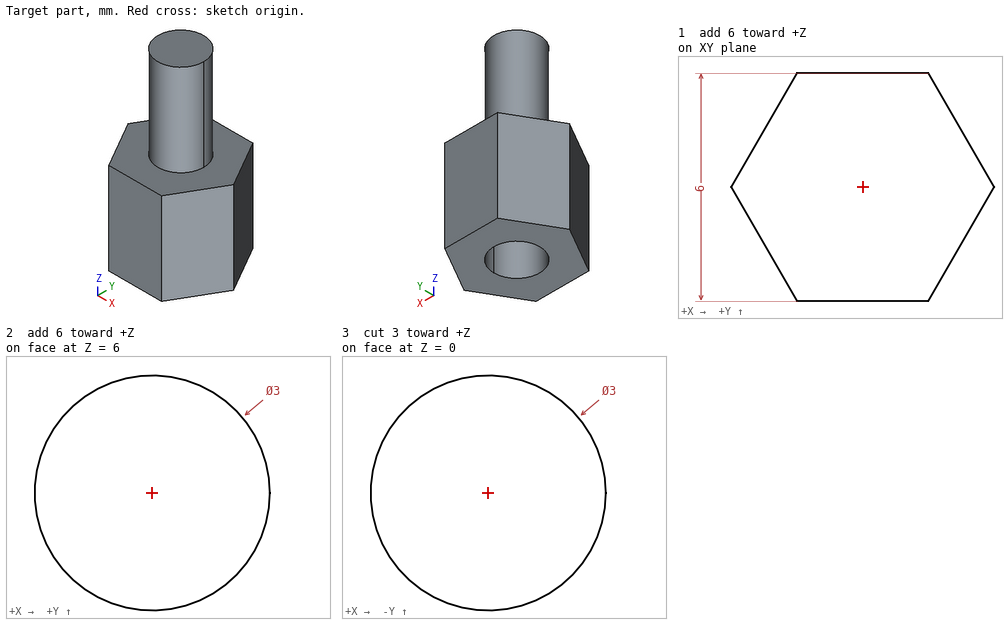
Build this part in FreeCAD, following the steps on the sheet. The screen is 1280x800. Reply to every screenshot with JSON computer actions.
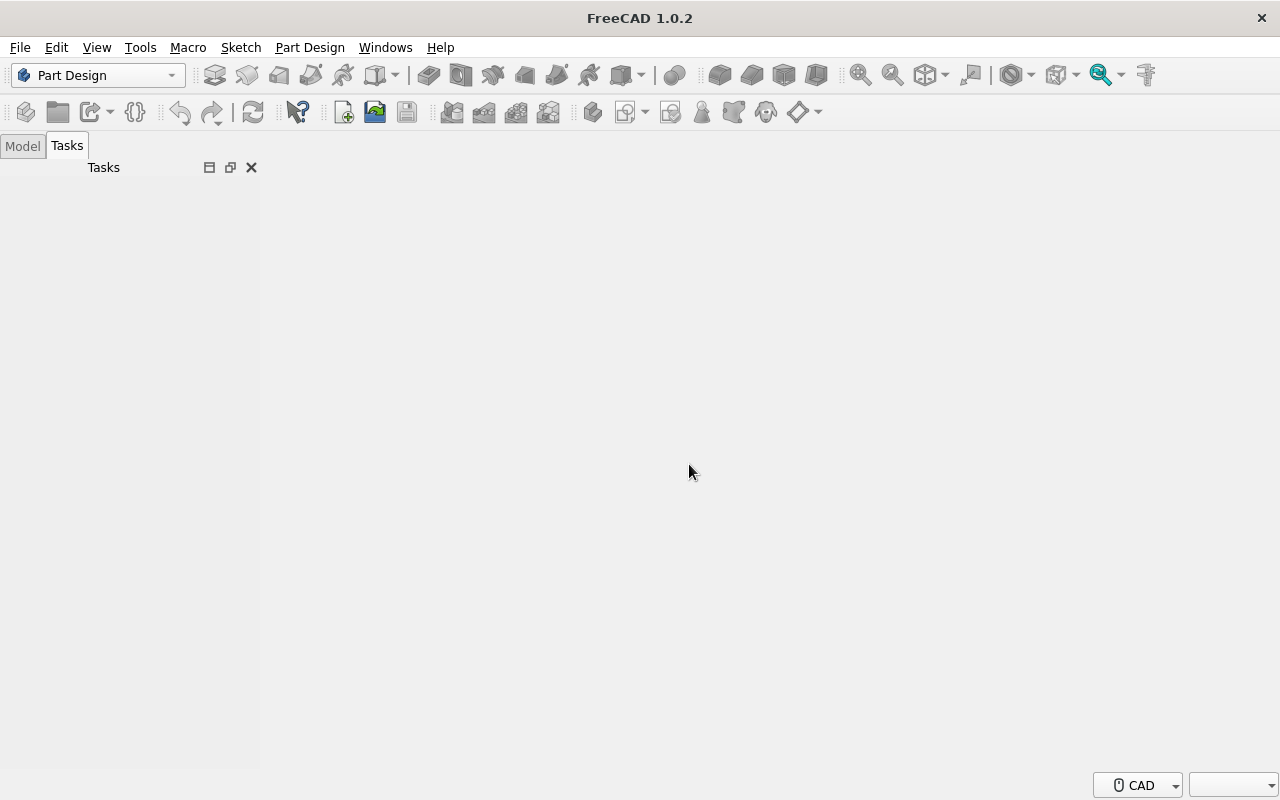
{"action": "left_click", "coordinate": [344, 112]}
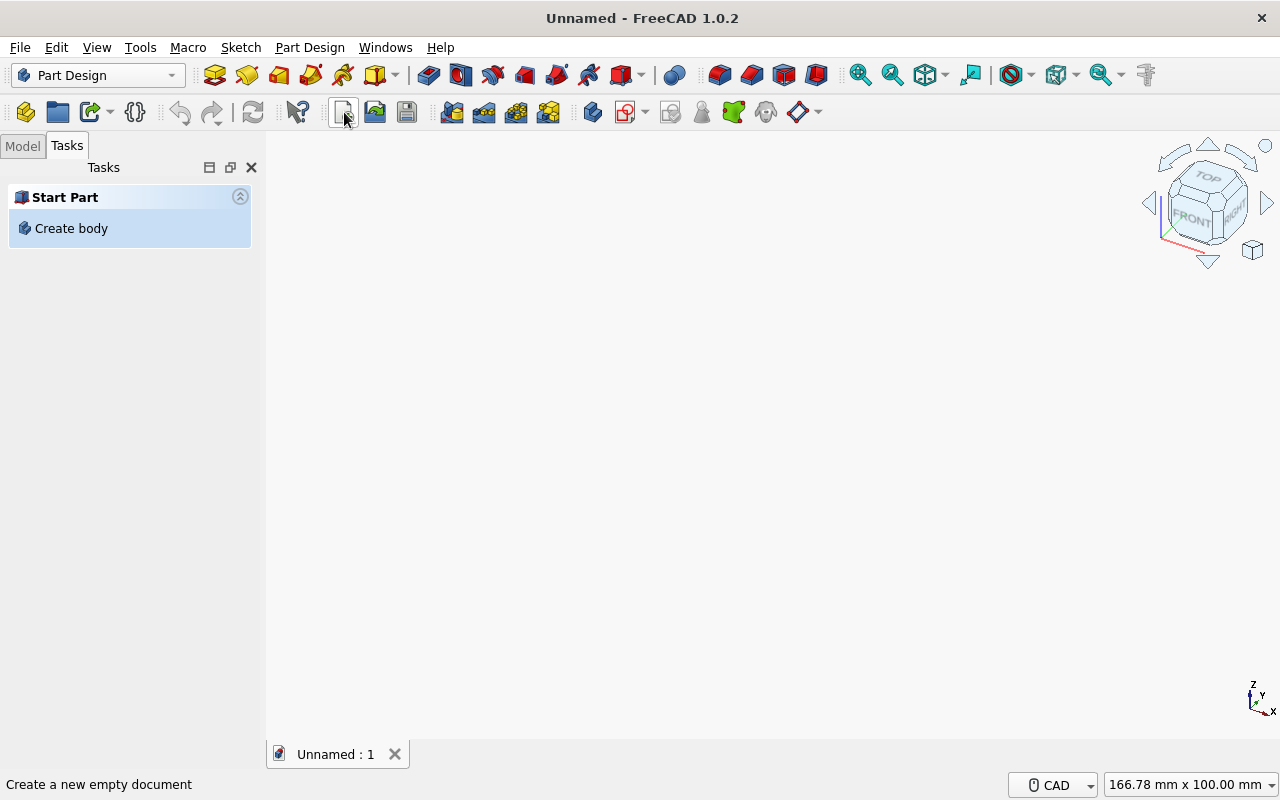
{"action": "left_click", "coordinate": [626, 112]}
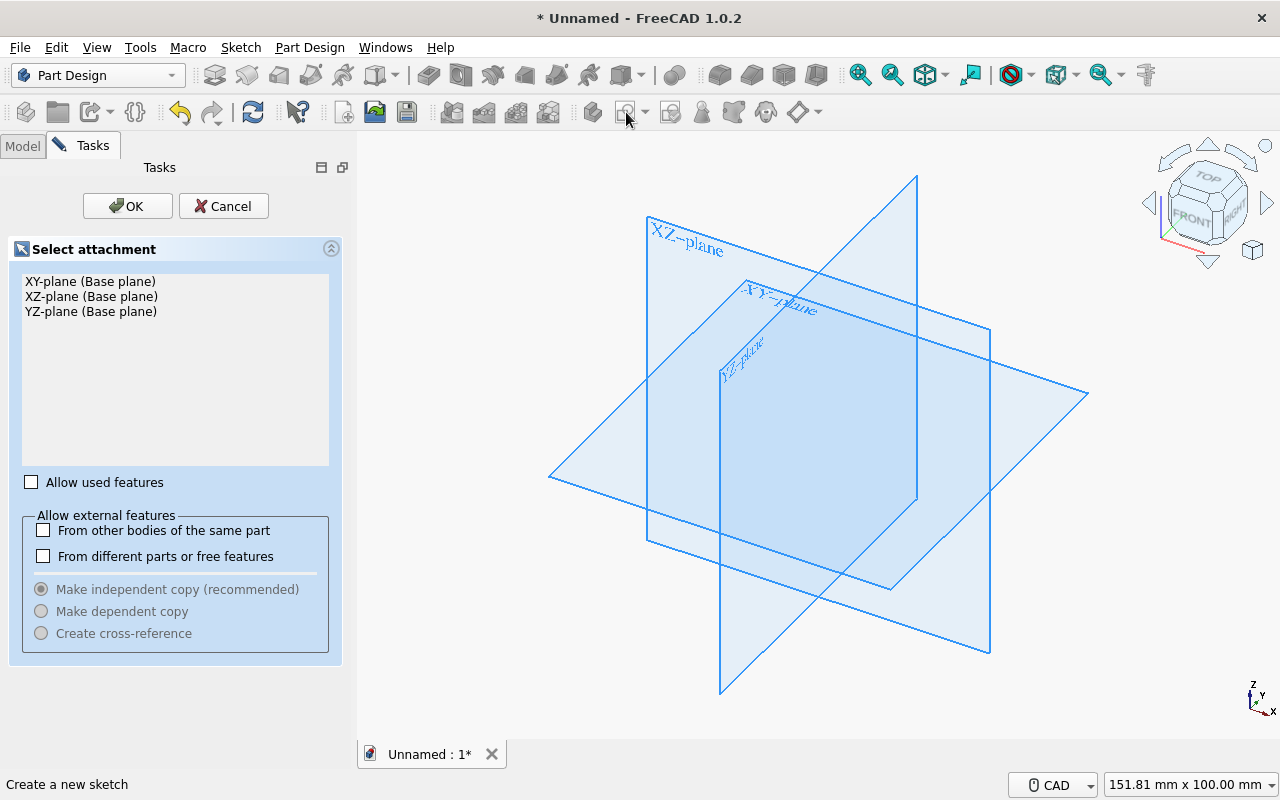
{"action": "left_click", "coordinate": [82, 282]}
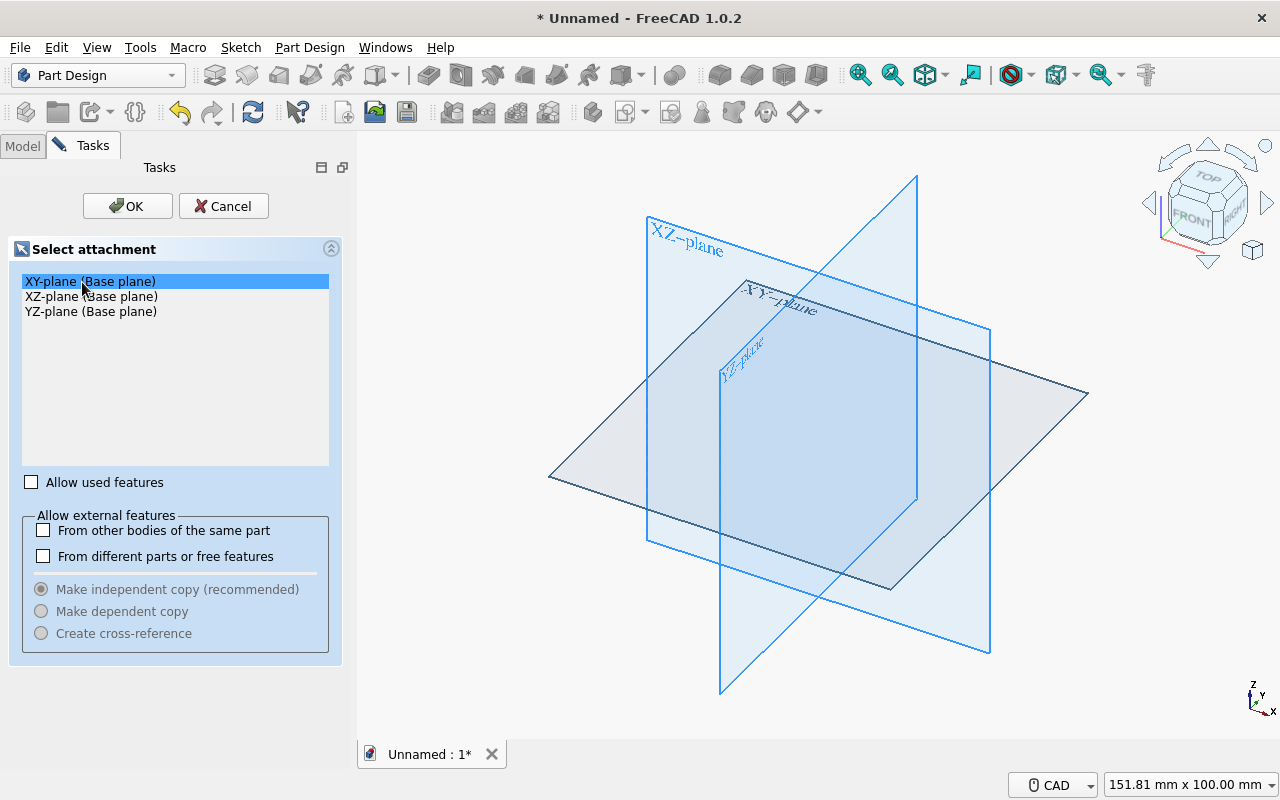
{"action": "left_click", "coordinate": [128, 206]}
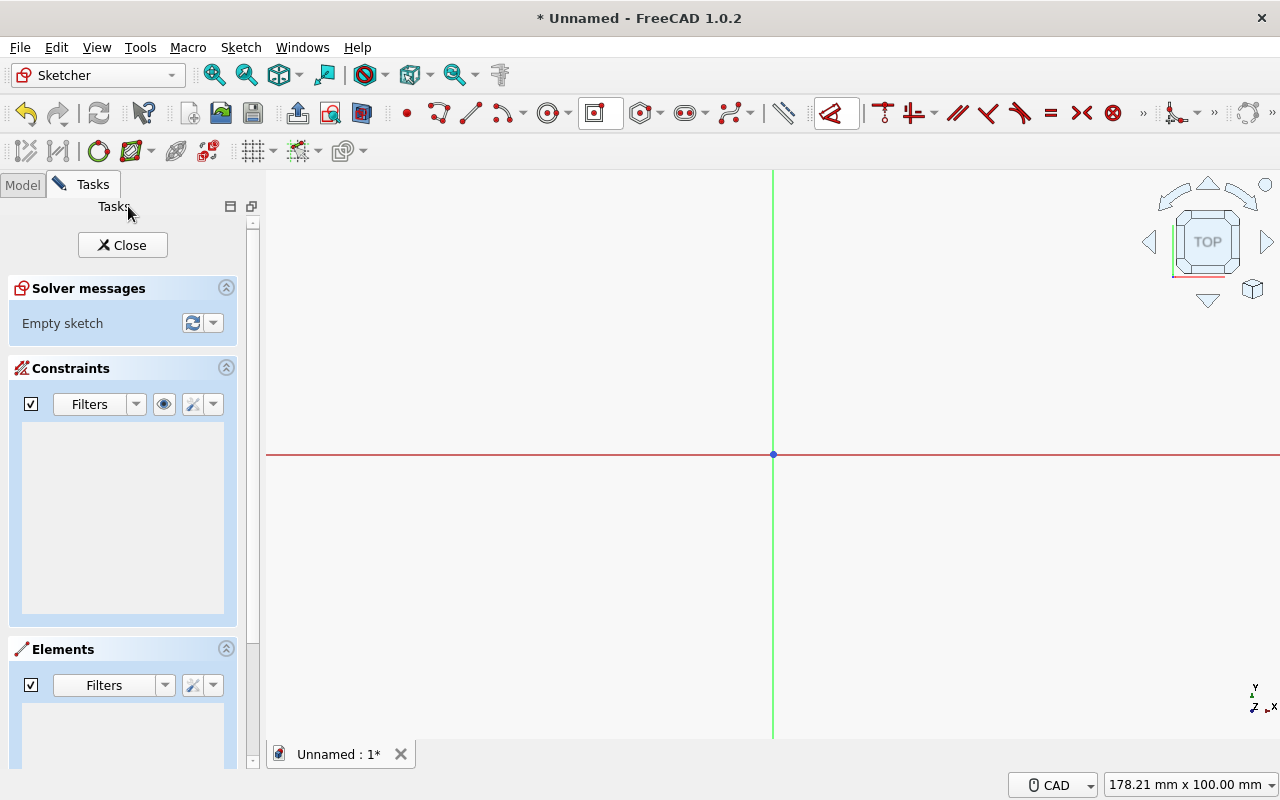
{"action": "scroll", "coordinate": [780, 455], "scroll_direction": "up", "scroll_amount": 12}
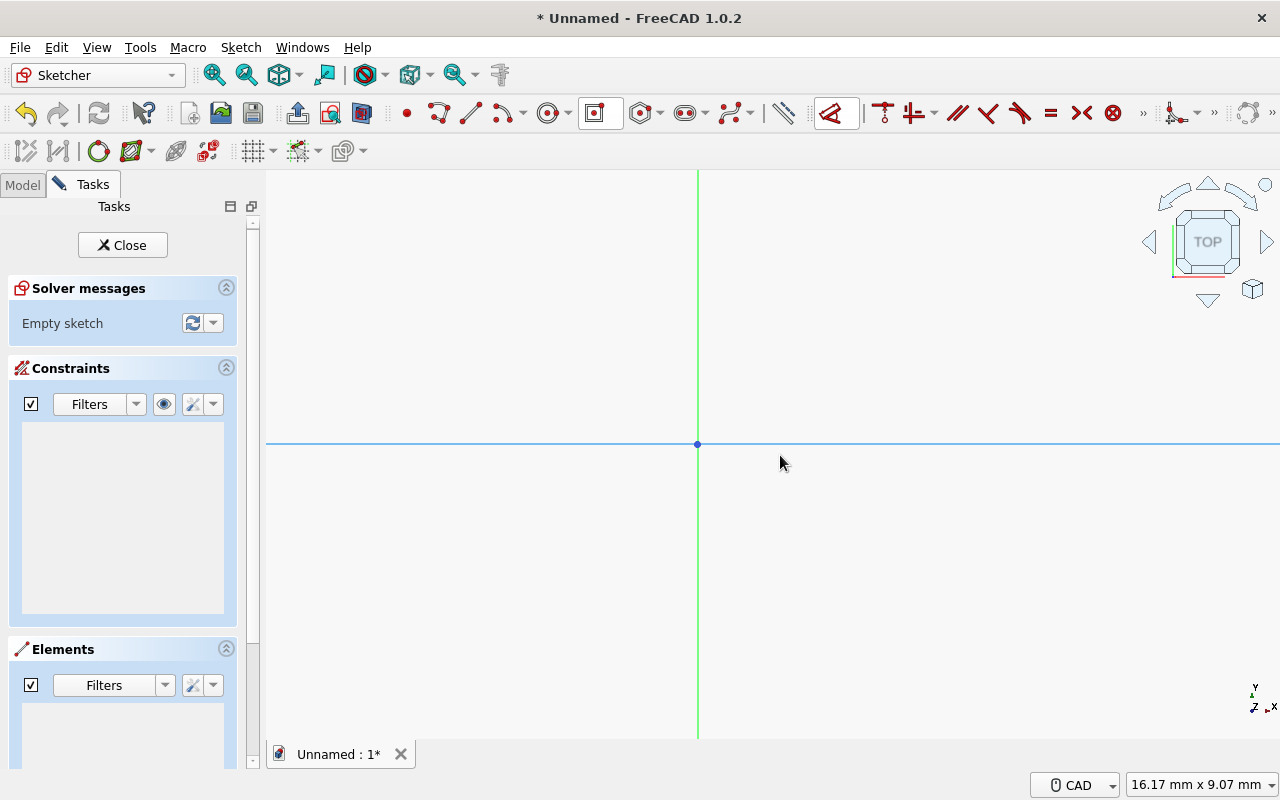
{"action": "key", "text": "g p 6"}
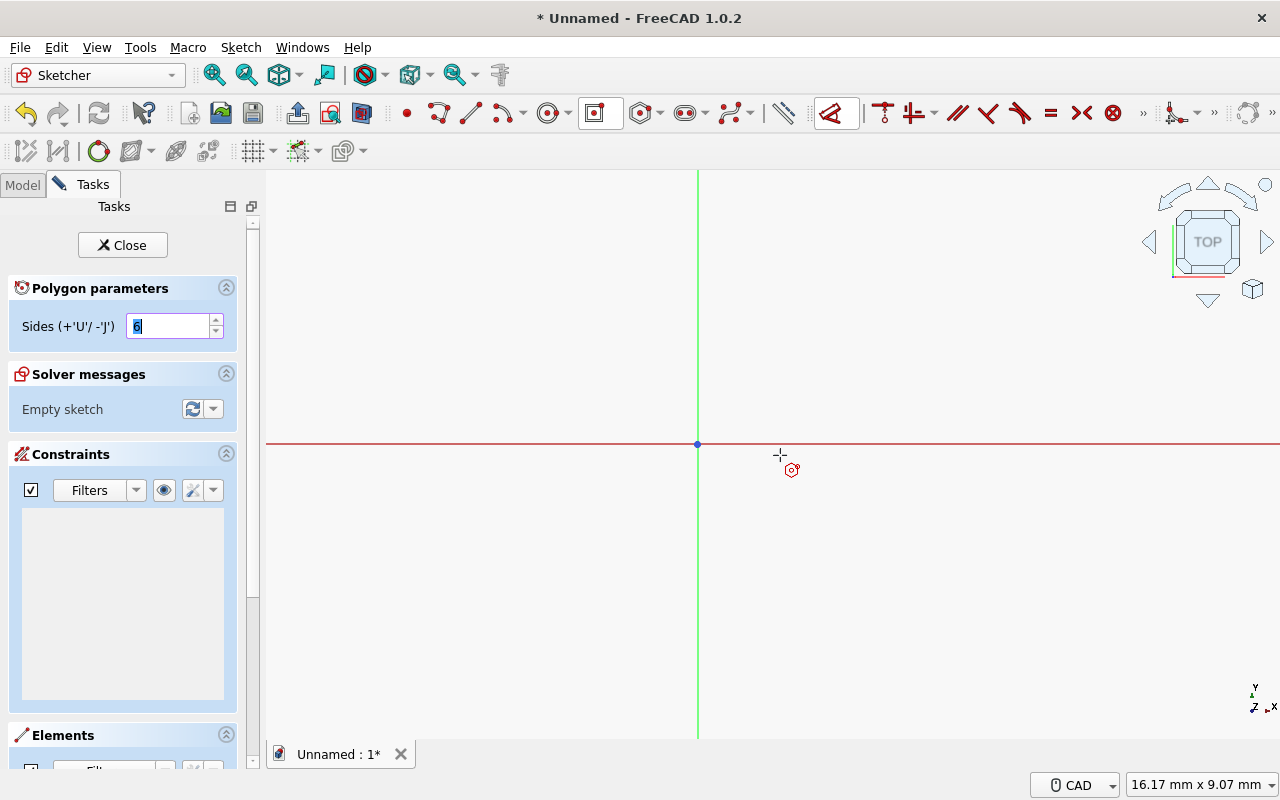
{"action": "left_click", "coordinate": [698, 444]}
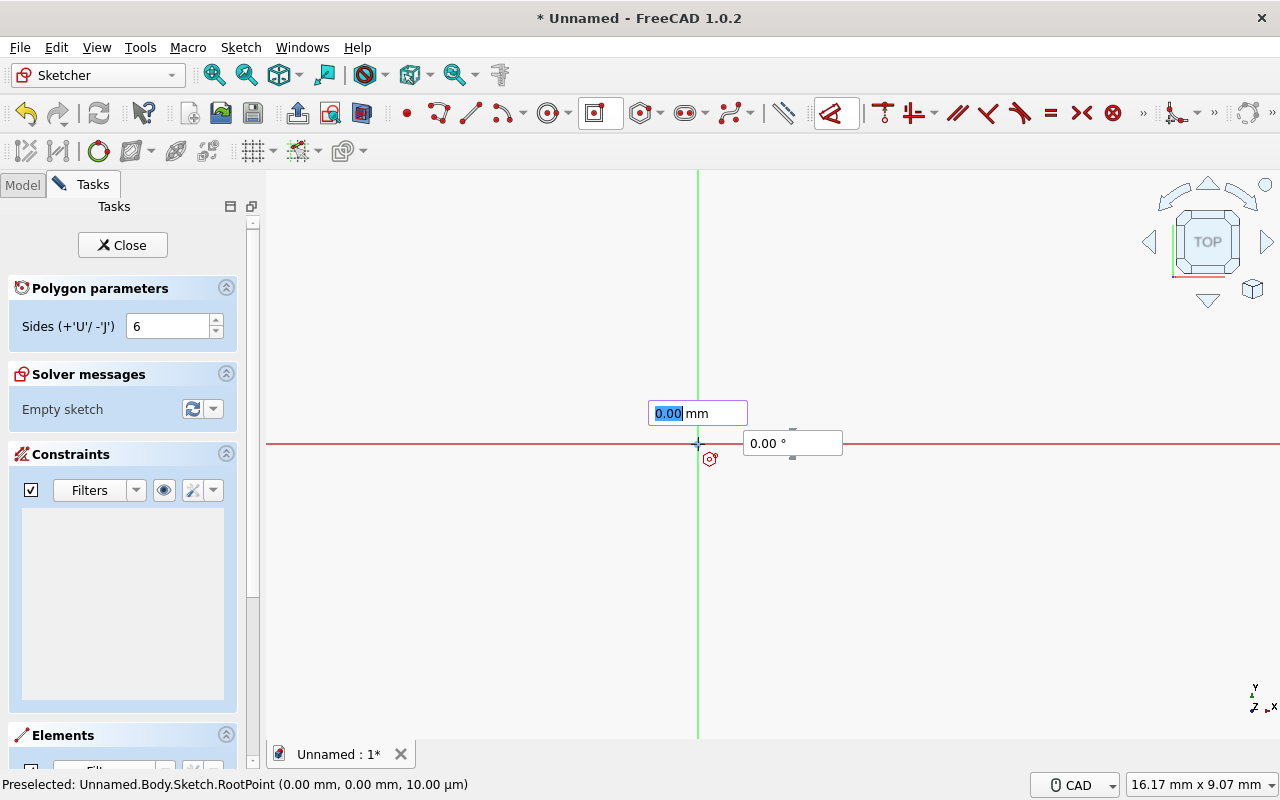
{"action": "left_click", "coordinate": [915, 444]}
{"action": "right_click", "coordinate": [915, 444]}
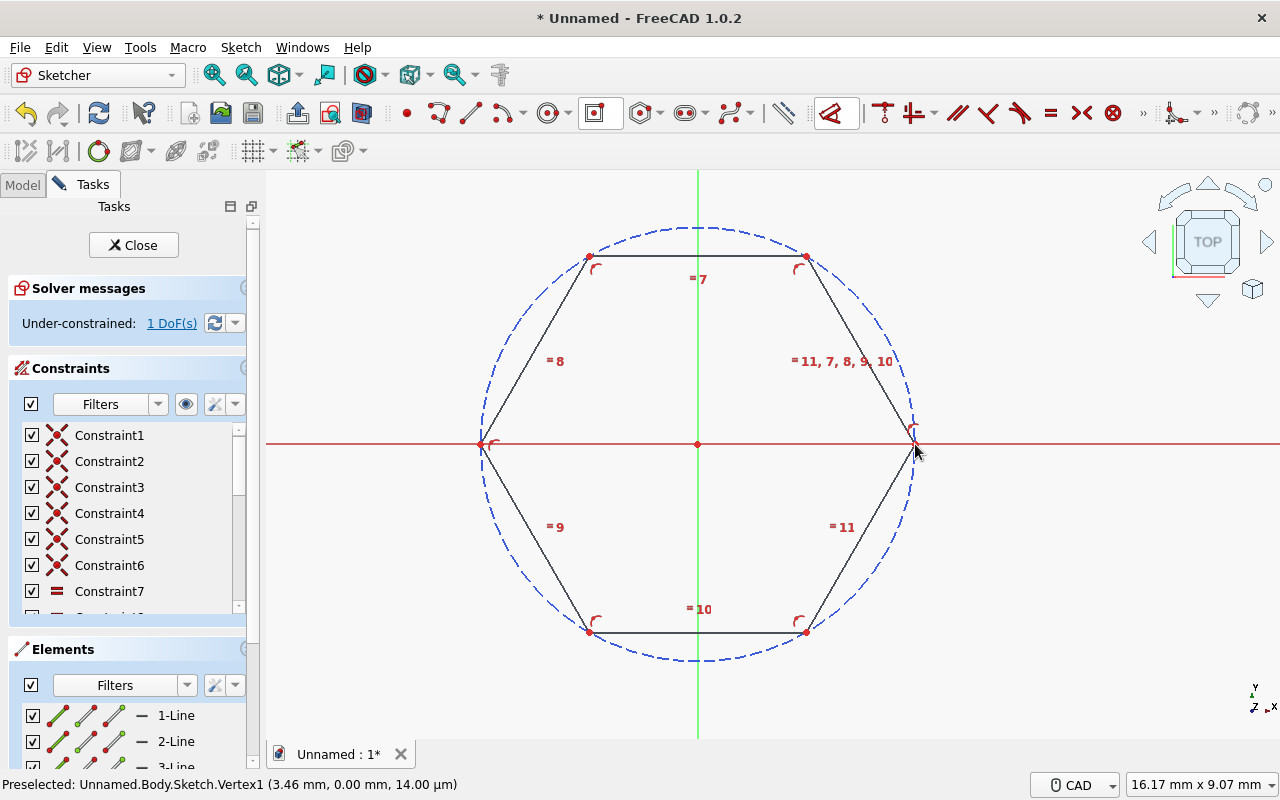
{"action": "left_click", "coordinate": [589, 633]}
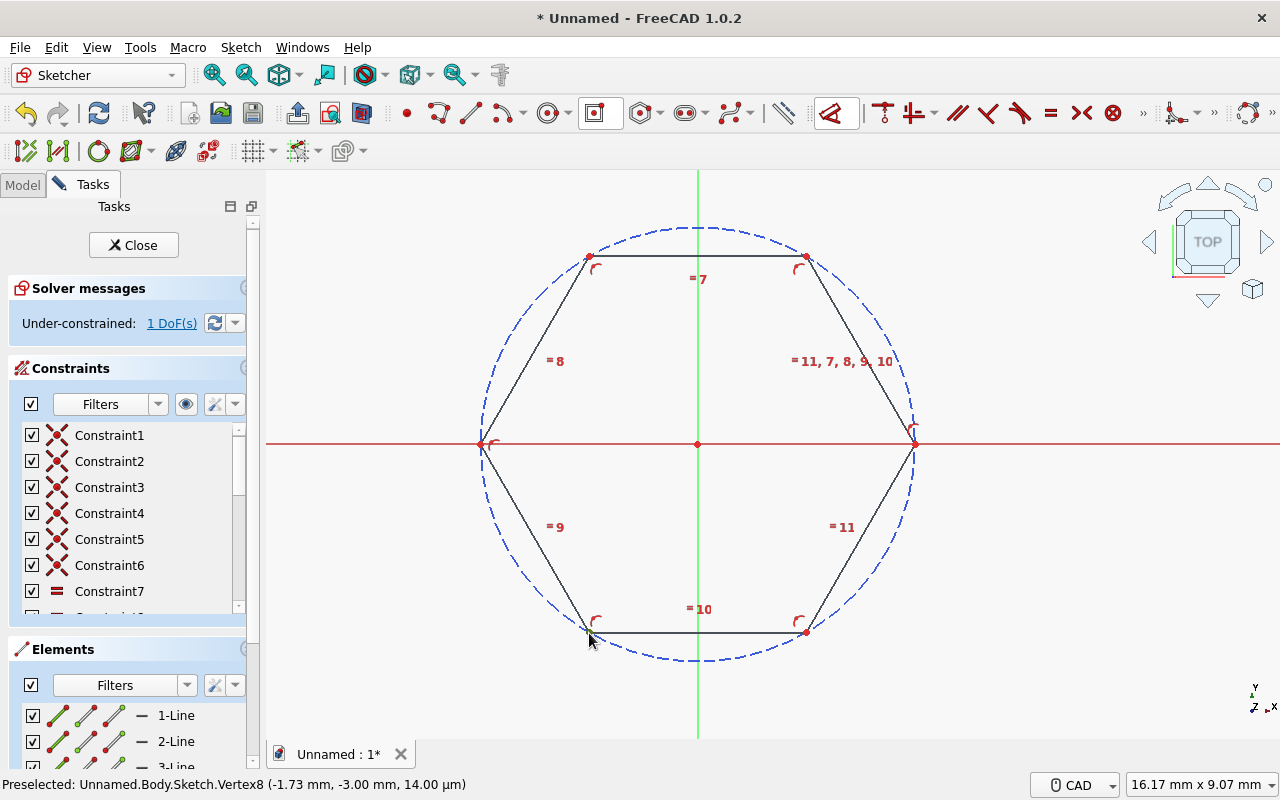
{"action": "left_click", "coordinate": [806, 256]}